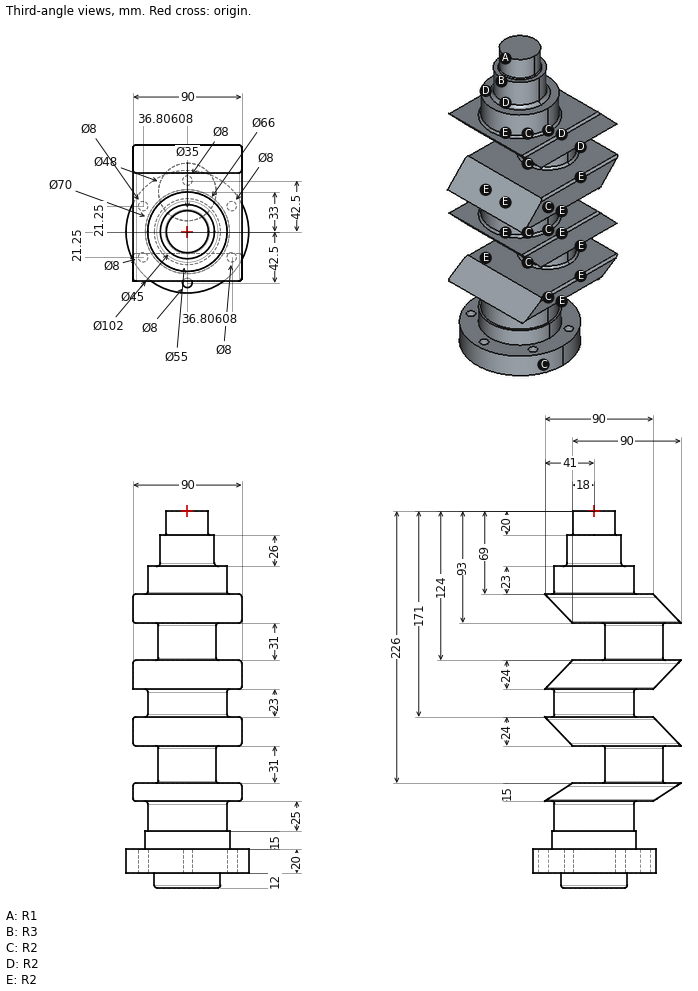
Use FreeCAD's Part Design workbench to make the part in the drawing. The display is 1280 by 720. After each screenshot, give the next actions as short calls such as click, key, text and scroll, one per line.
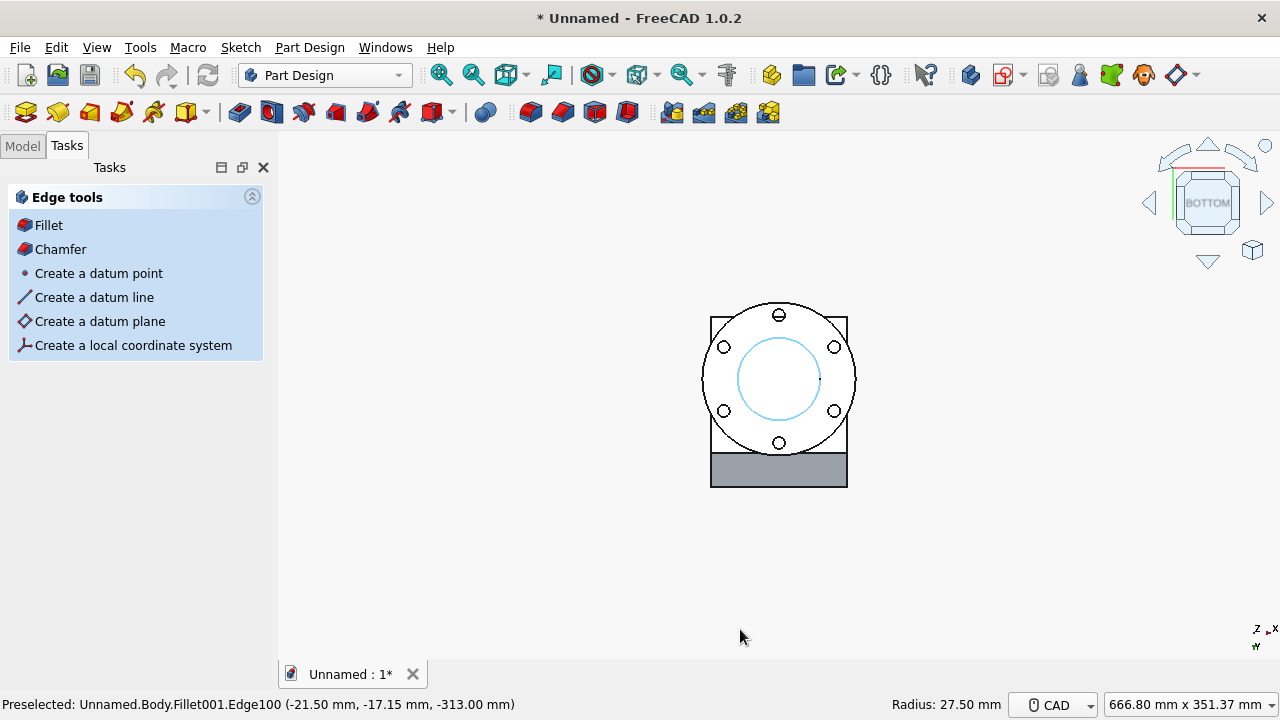
click(442, 76)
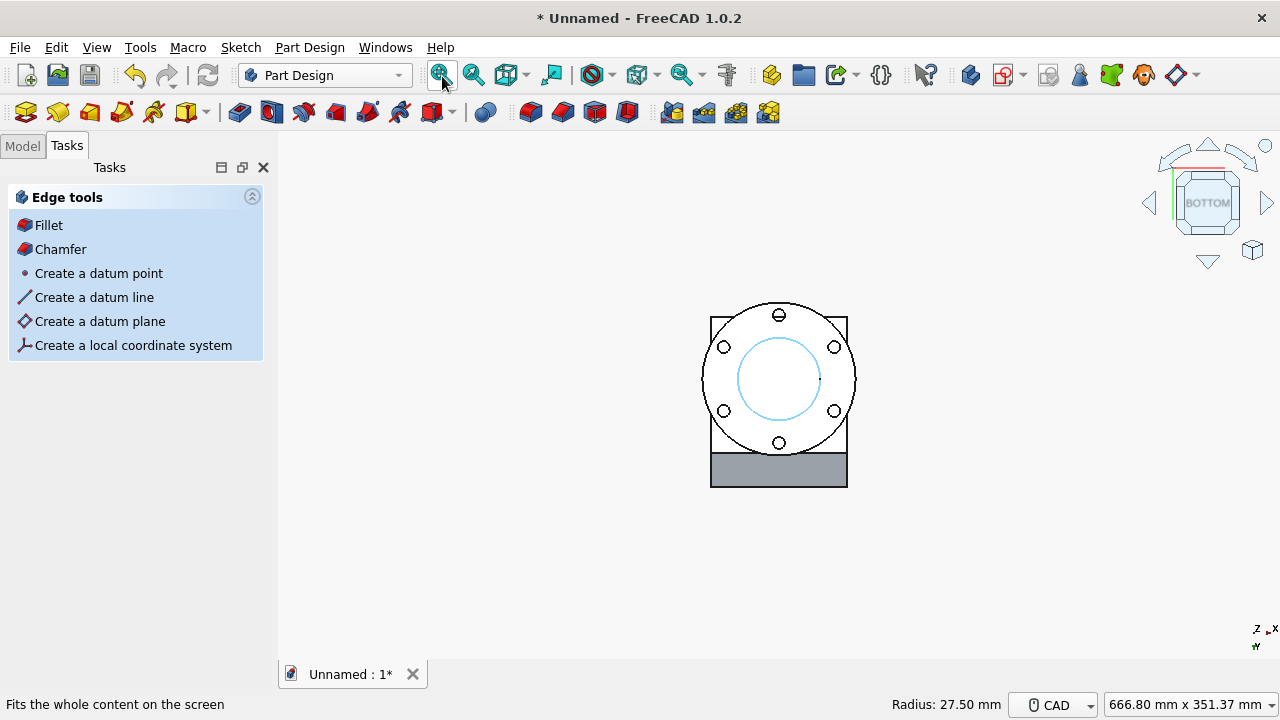
key(4)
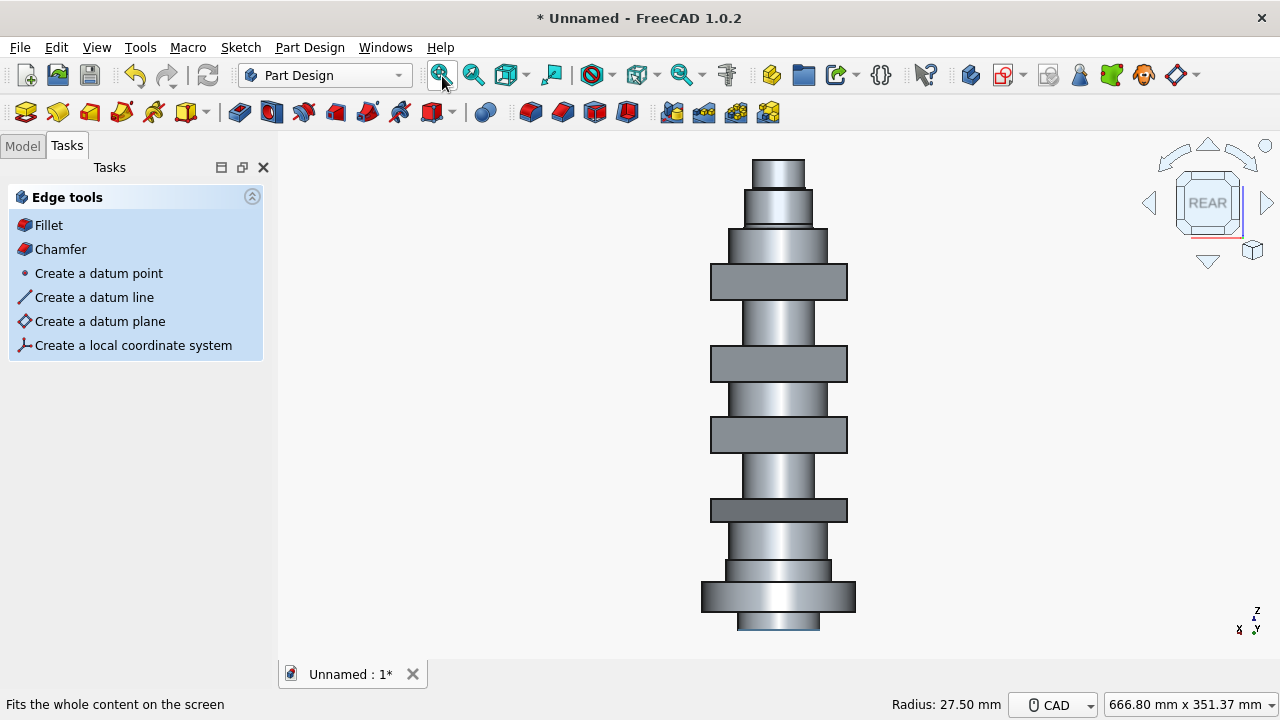
key(6)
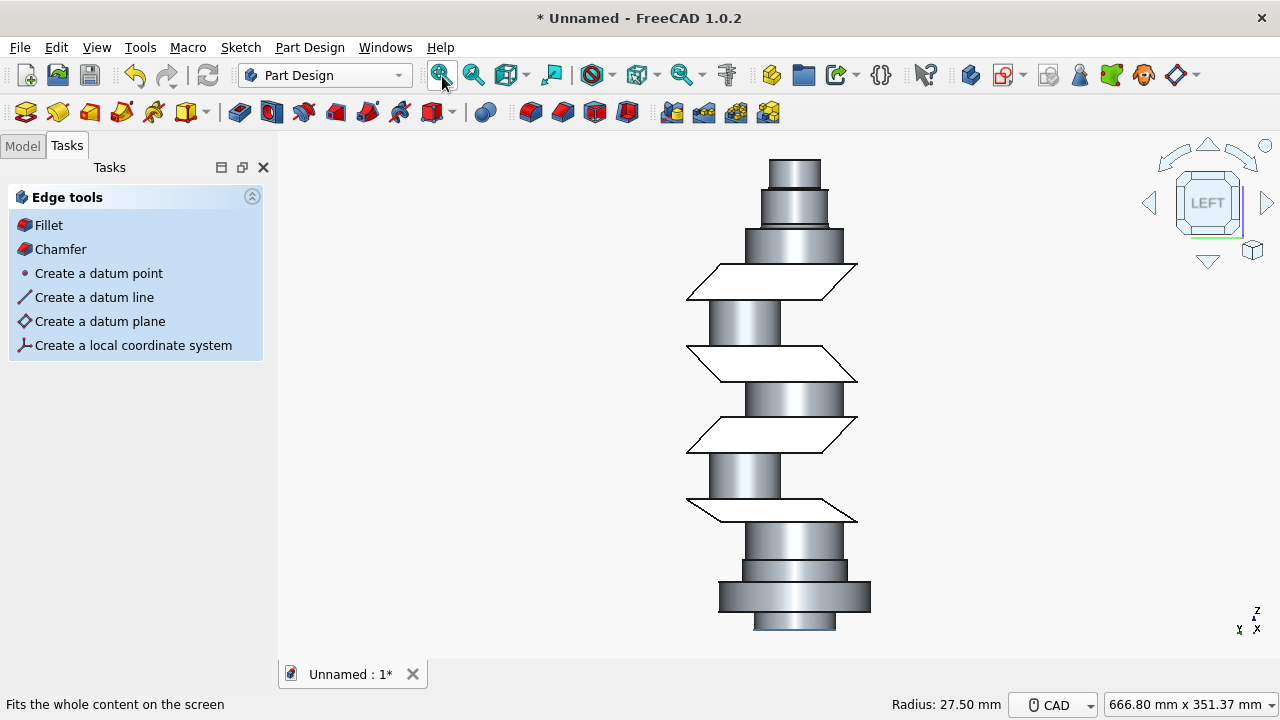
key(v)
key(3)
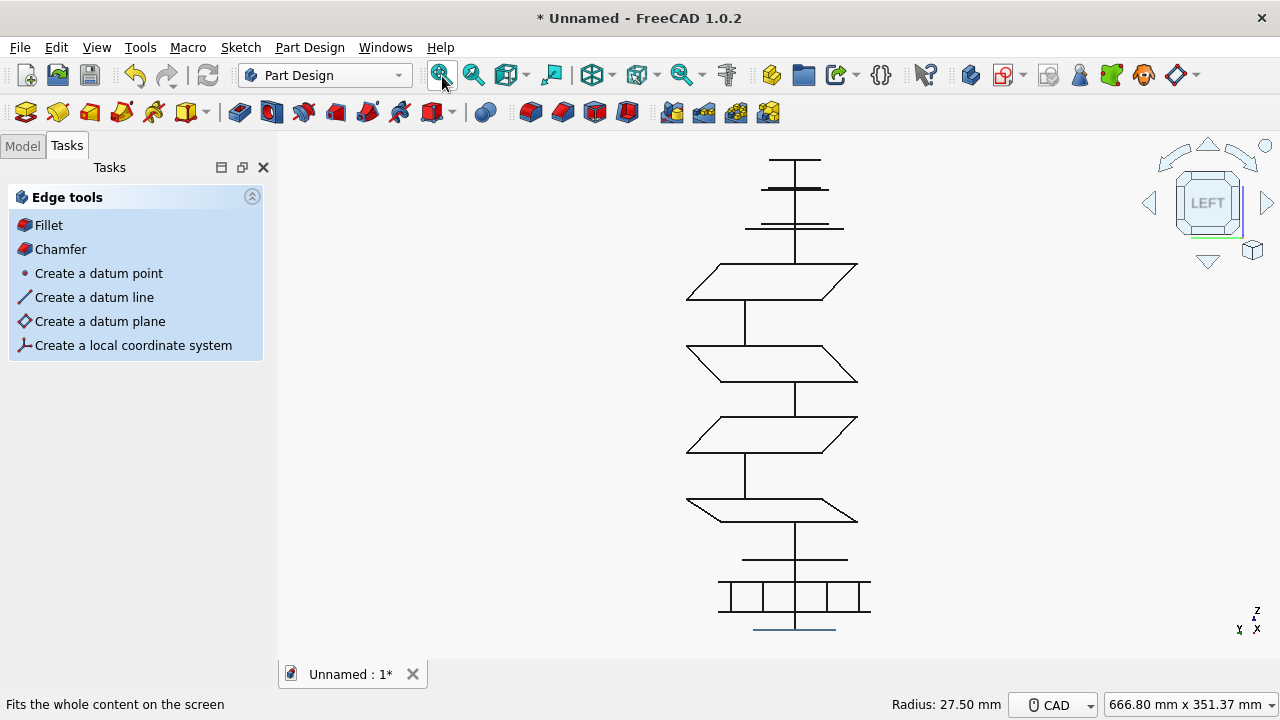
key(0)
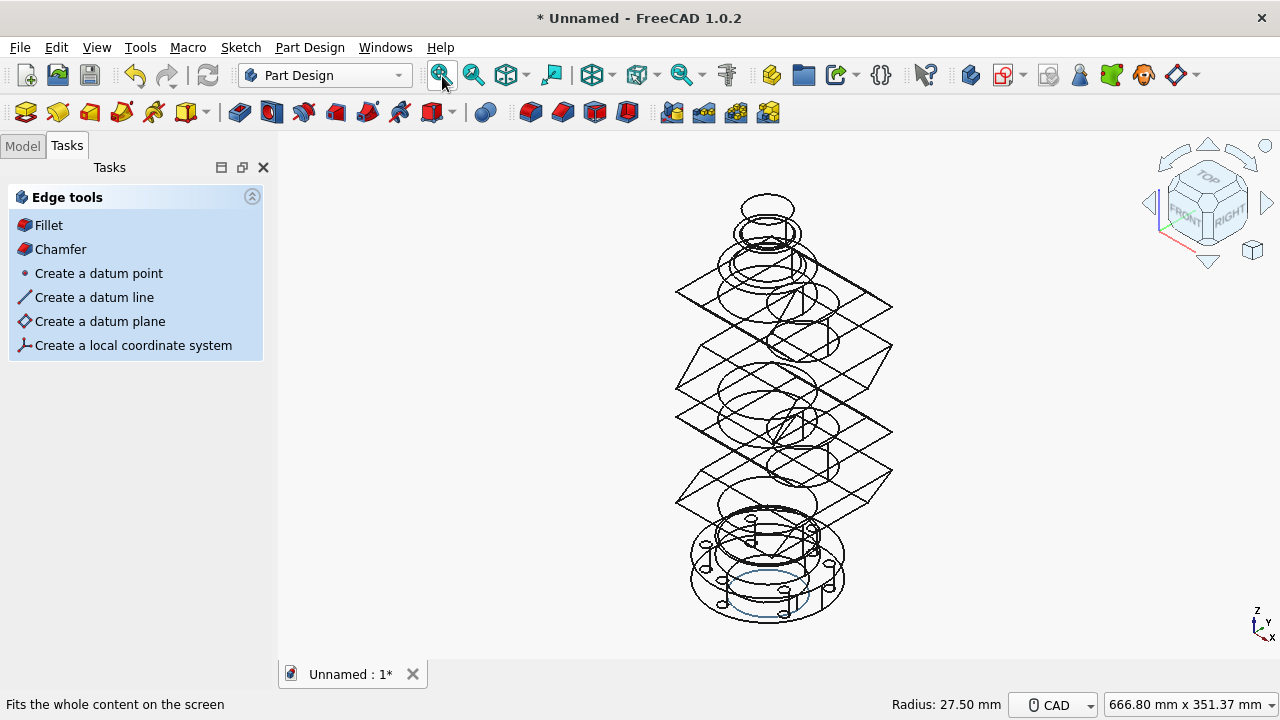
click(719, 289, ctrl)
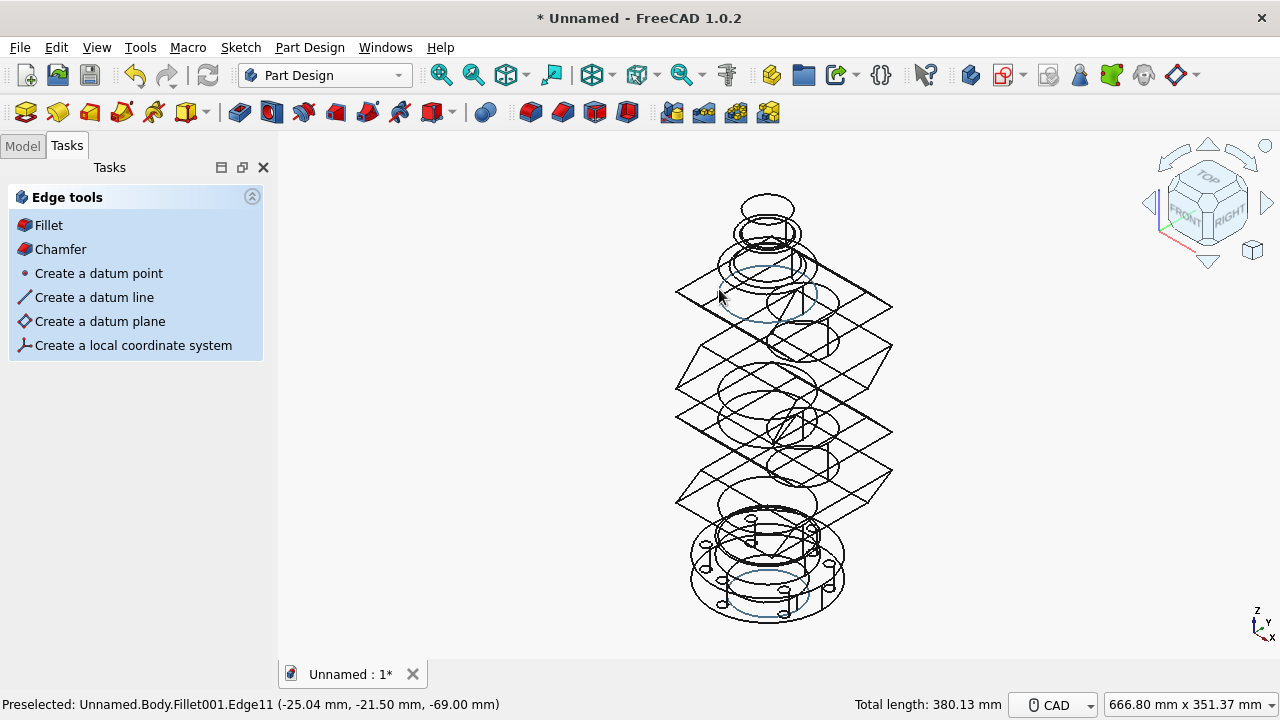
click(771, 312, ctrl)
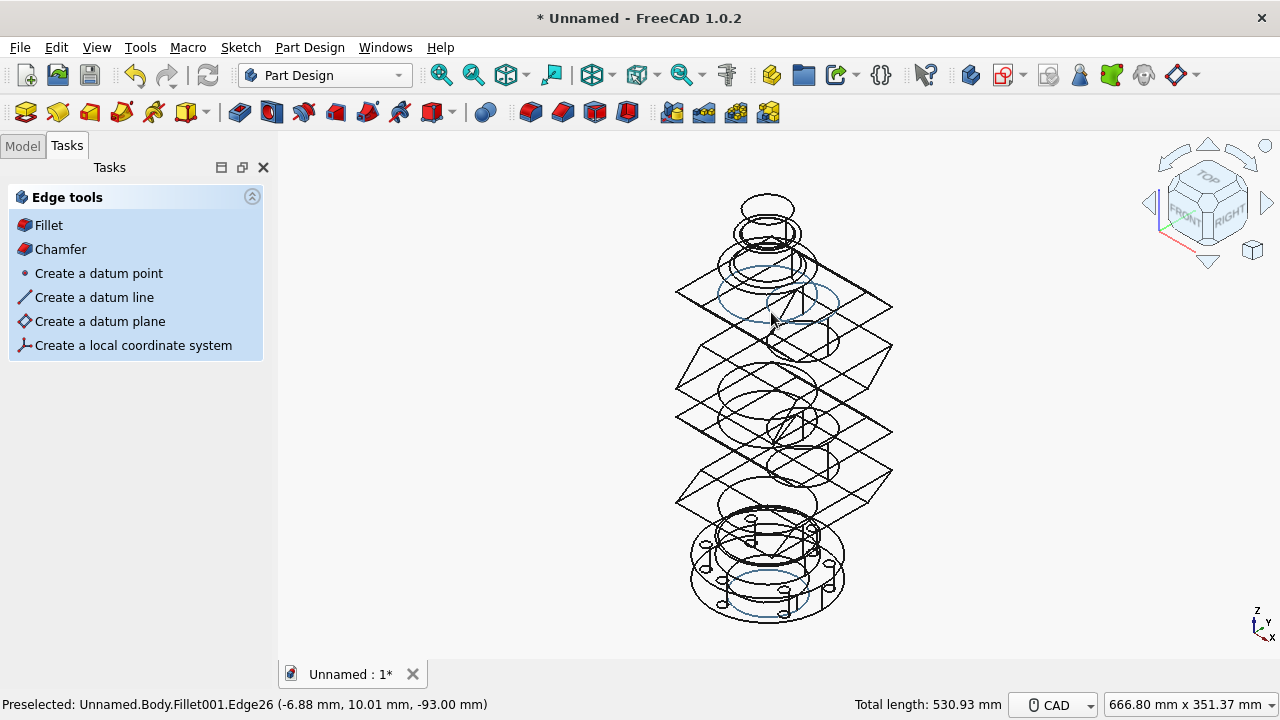
click(835, 331, ctrl)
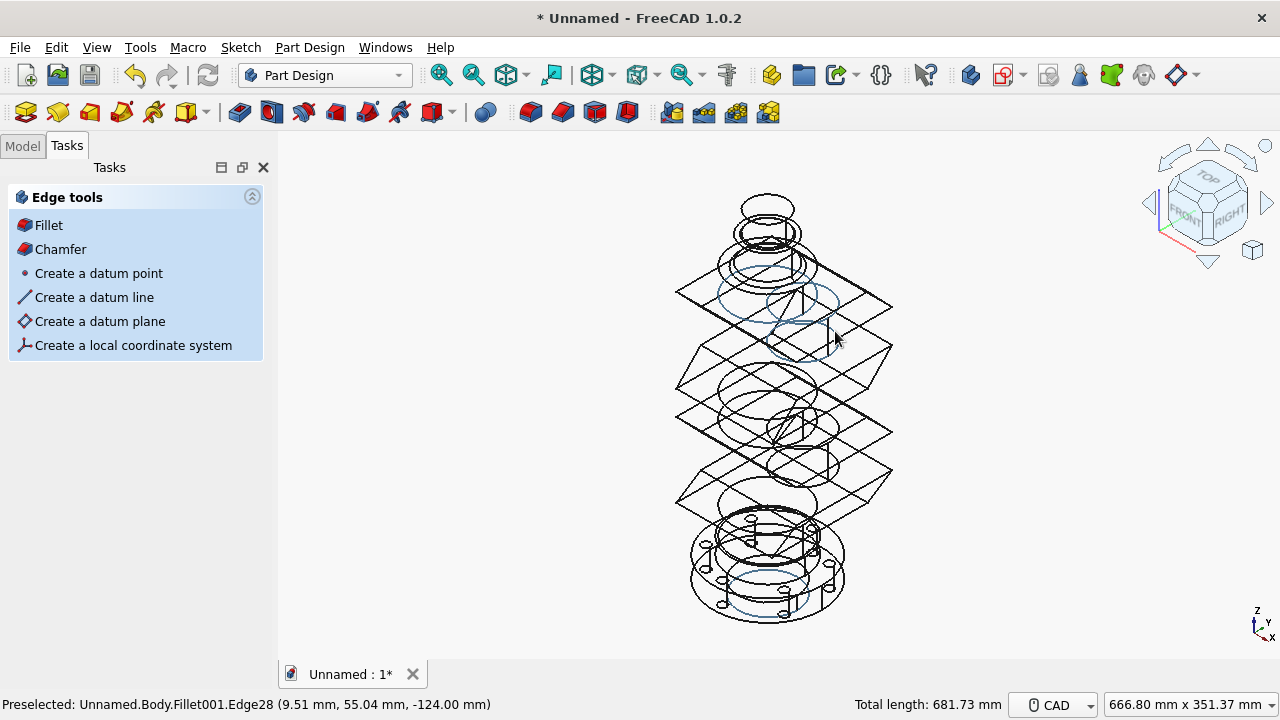
click(733, 370, ctrl)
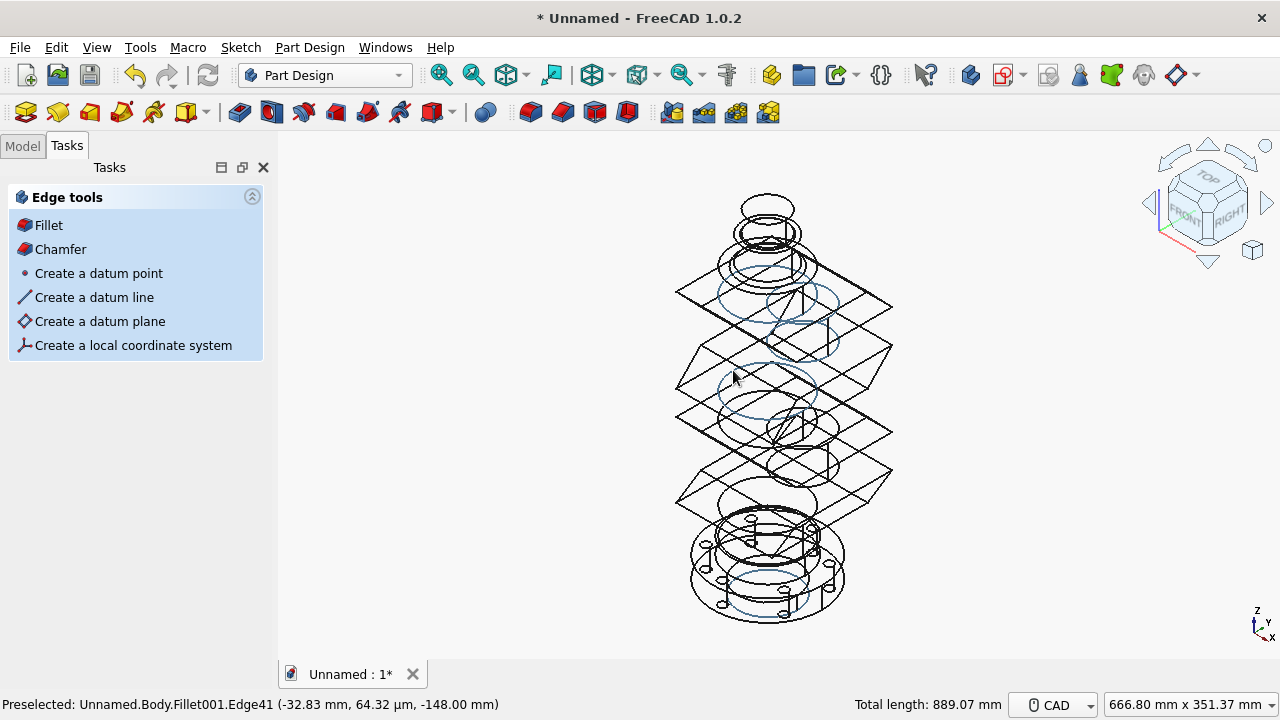
click(733, 398, ctrl)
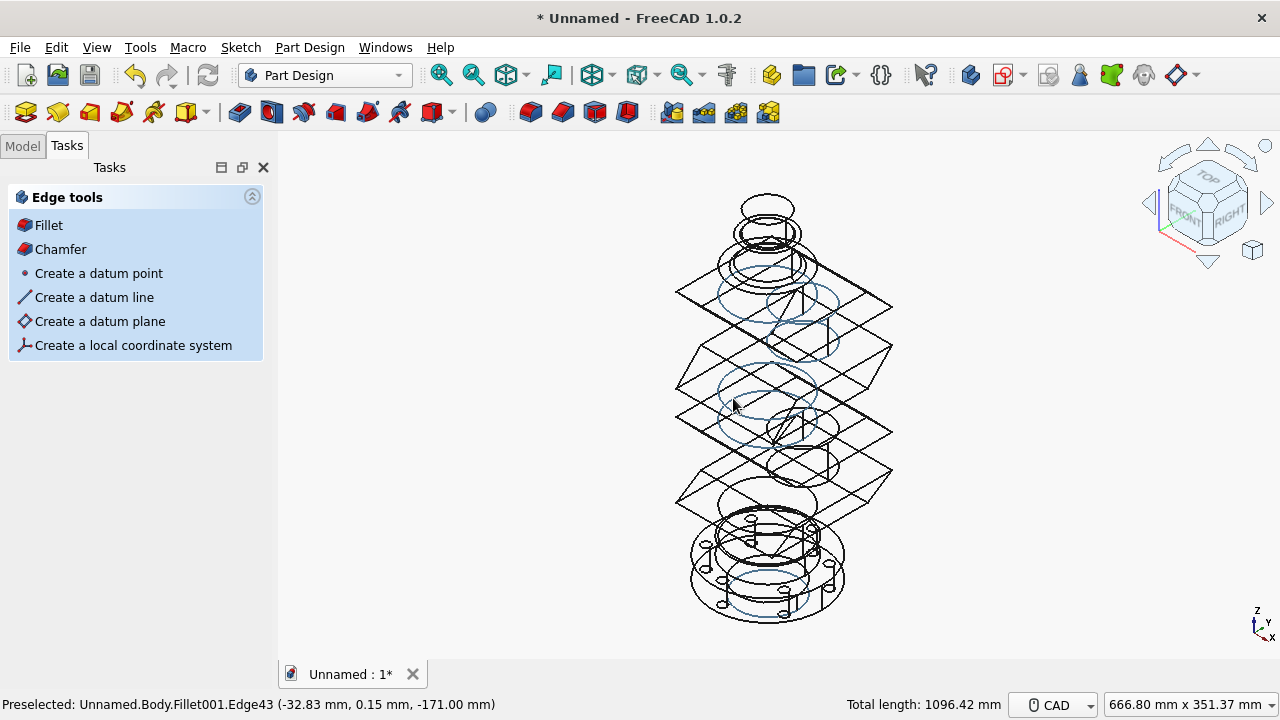
click(835, 418, ctrl)